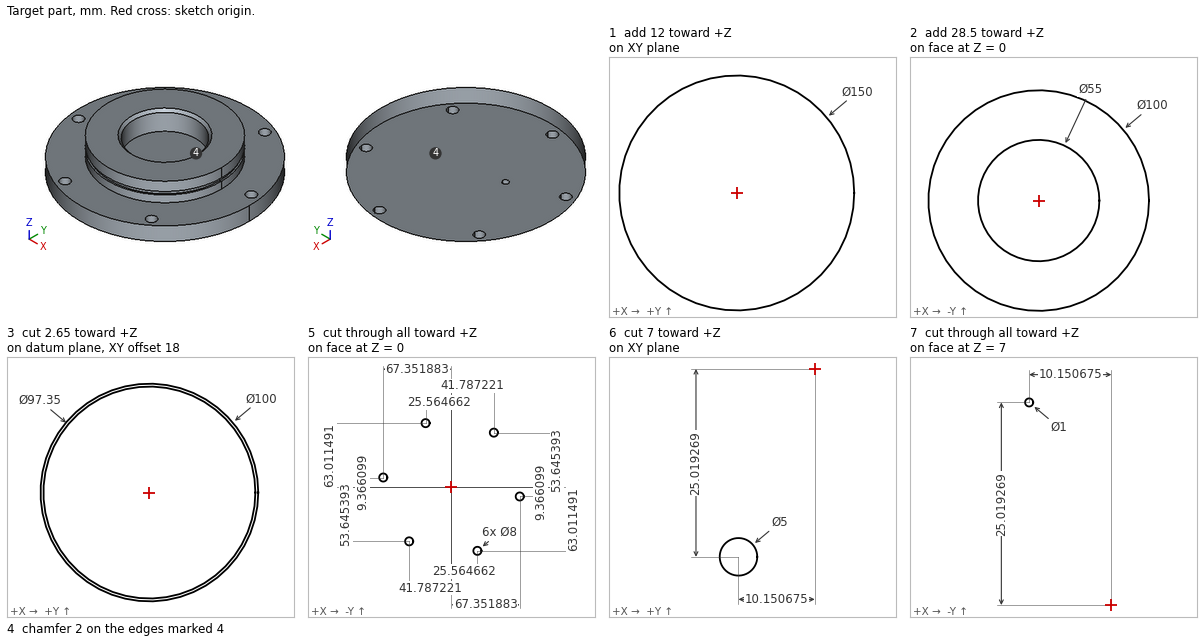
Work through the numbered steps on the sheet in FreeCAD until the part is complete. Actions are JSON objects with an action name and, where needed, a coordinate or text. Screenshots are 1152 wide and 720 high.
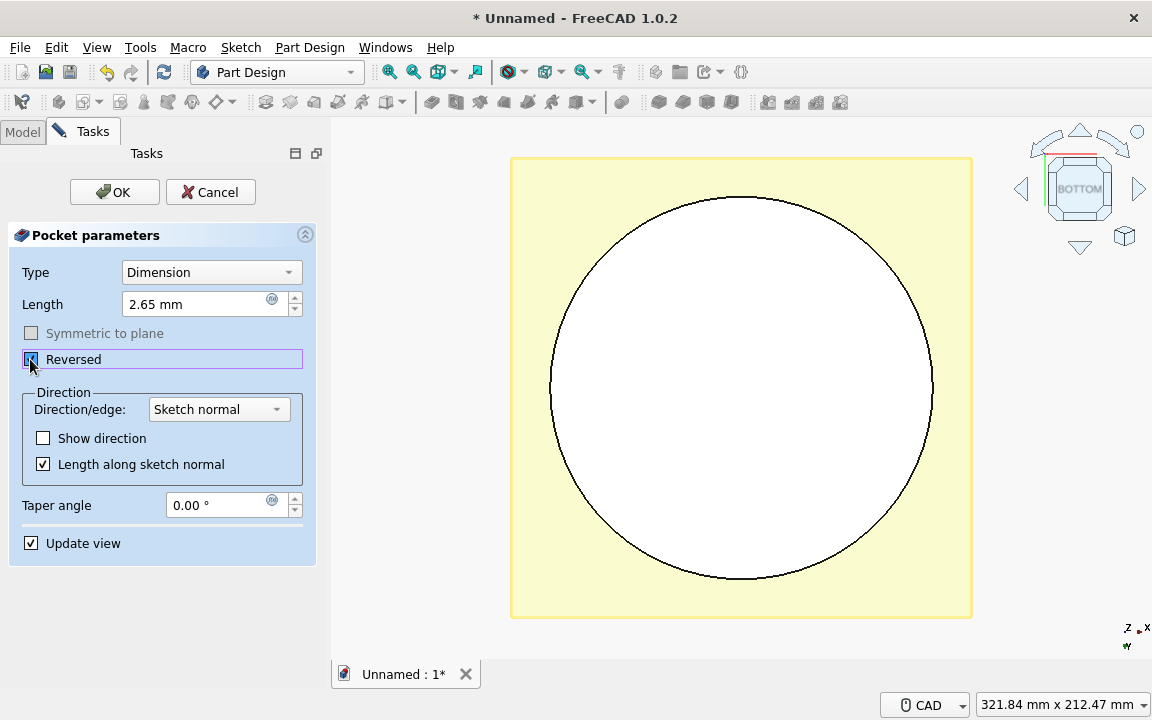
{"action": "left_click", "coordinate": [115, 192]}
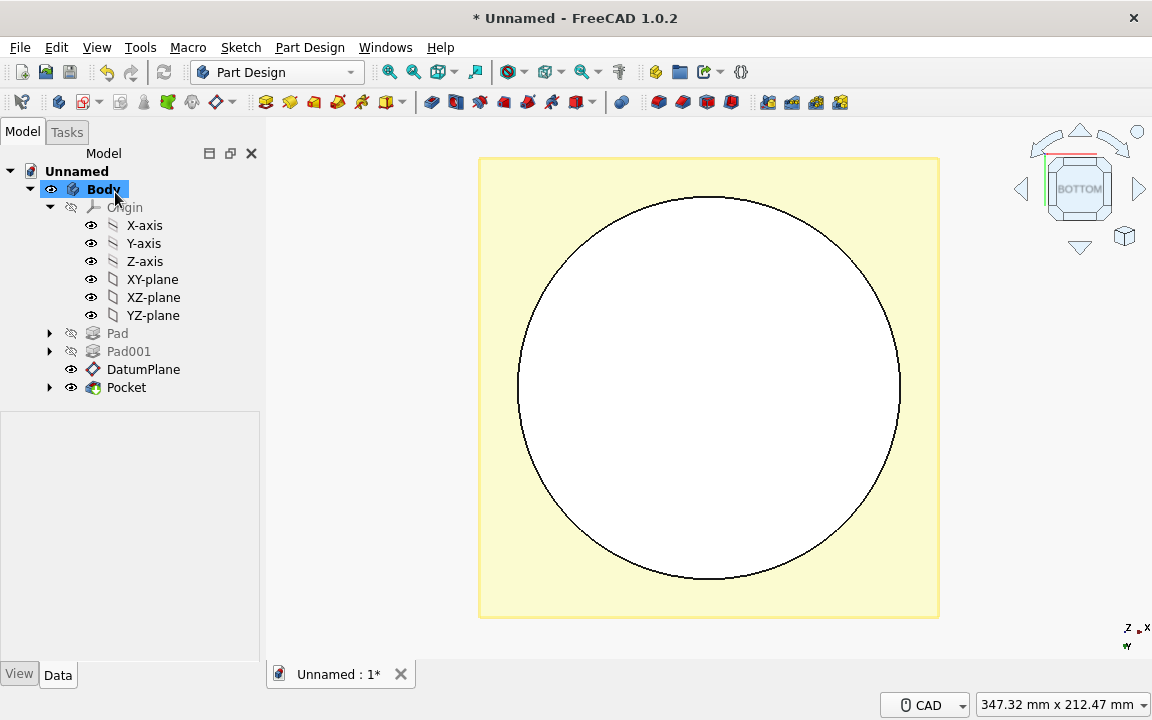
{"action": "left_click", "coordinate": [116, 369]}
{"action": "key", "text": "space"}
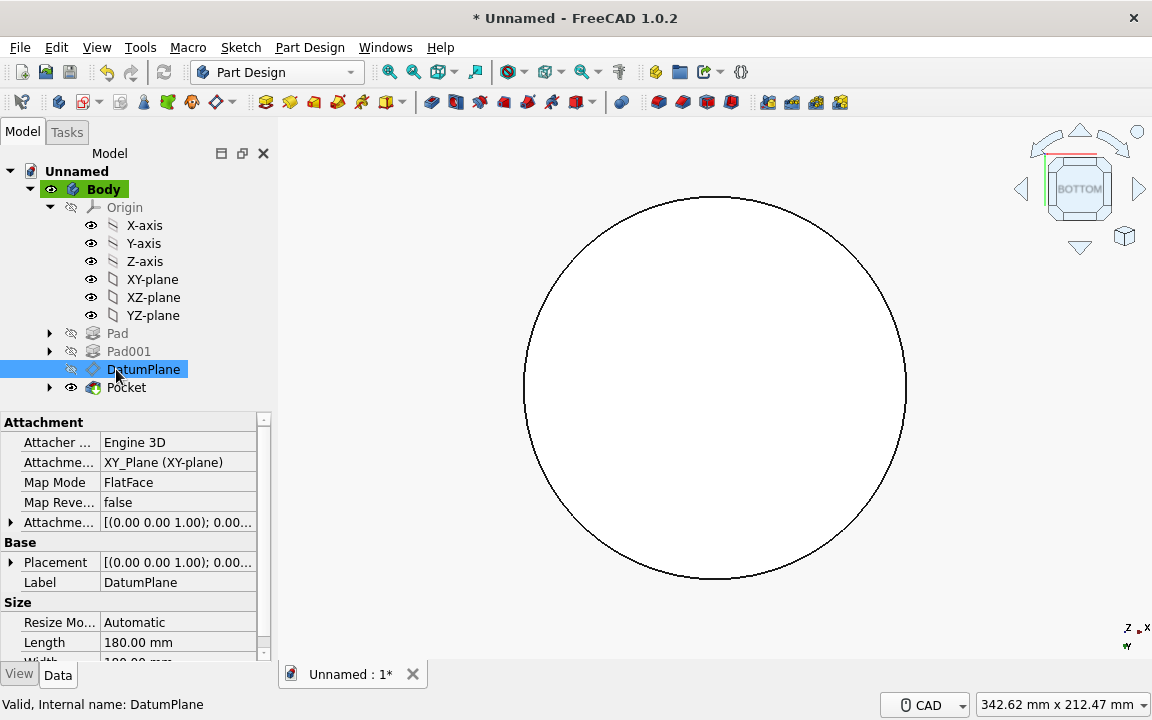
{"action": "key", "text": "0"}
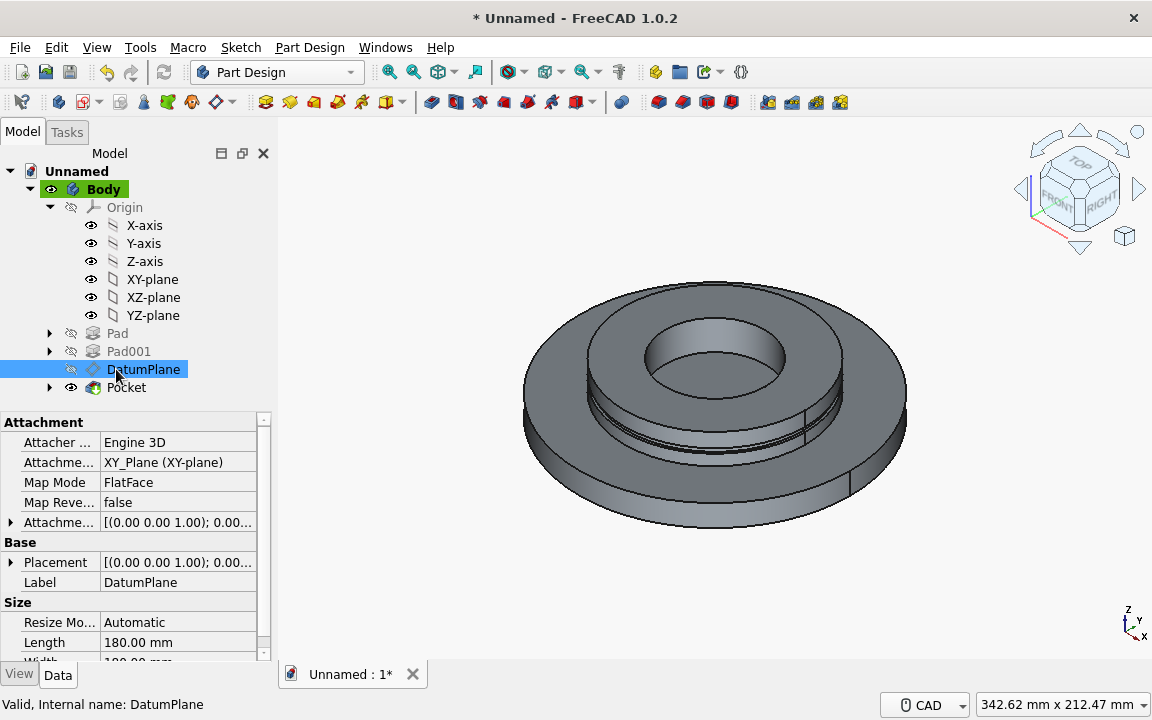
{"action": "left_click", "coordinate": [665, 329]}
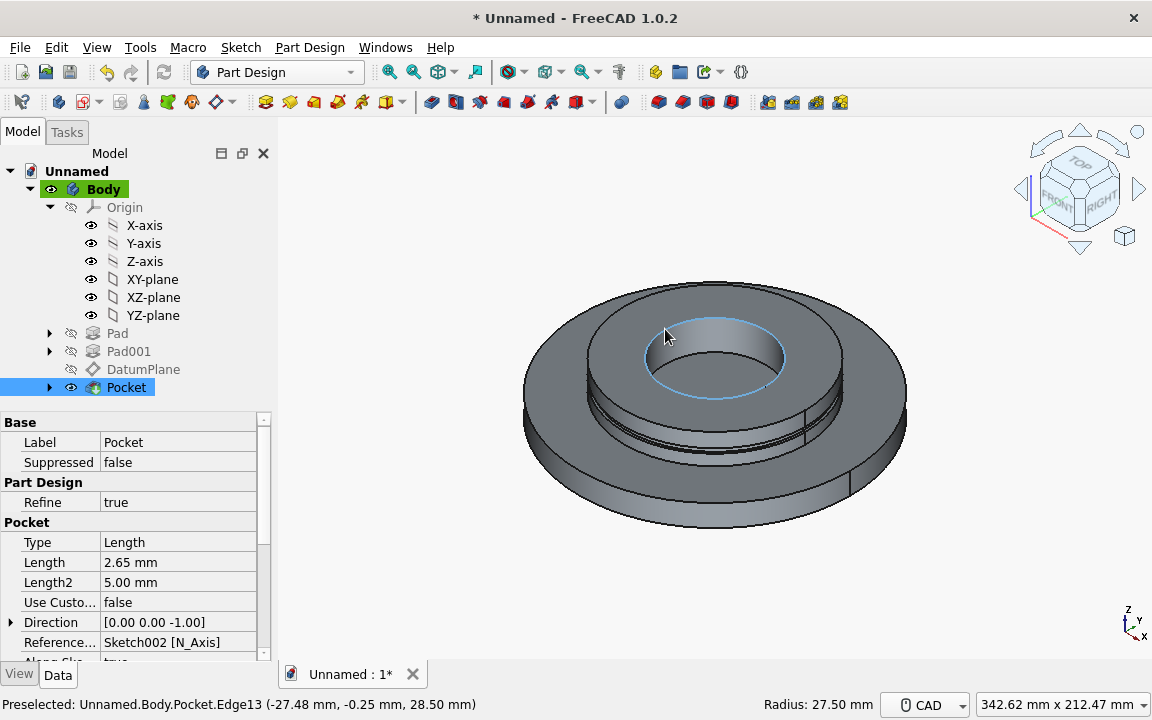
{"action": "left_click", "coordinate": [684, 102]}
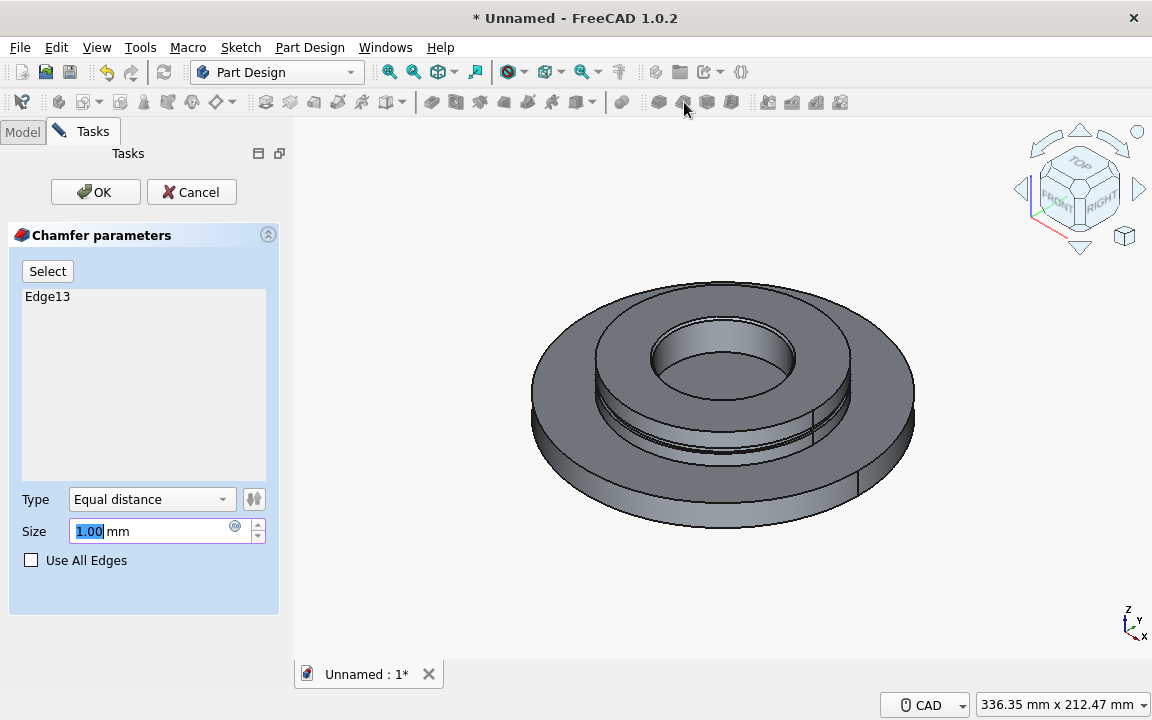
{"action": "type", "text": "2"}
{"action": "key", "text": "Tab"}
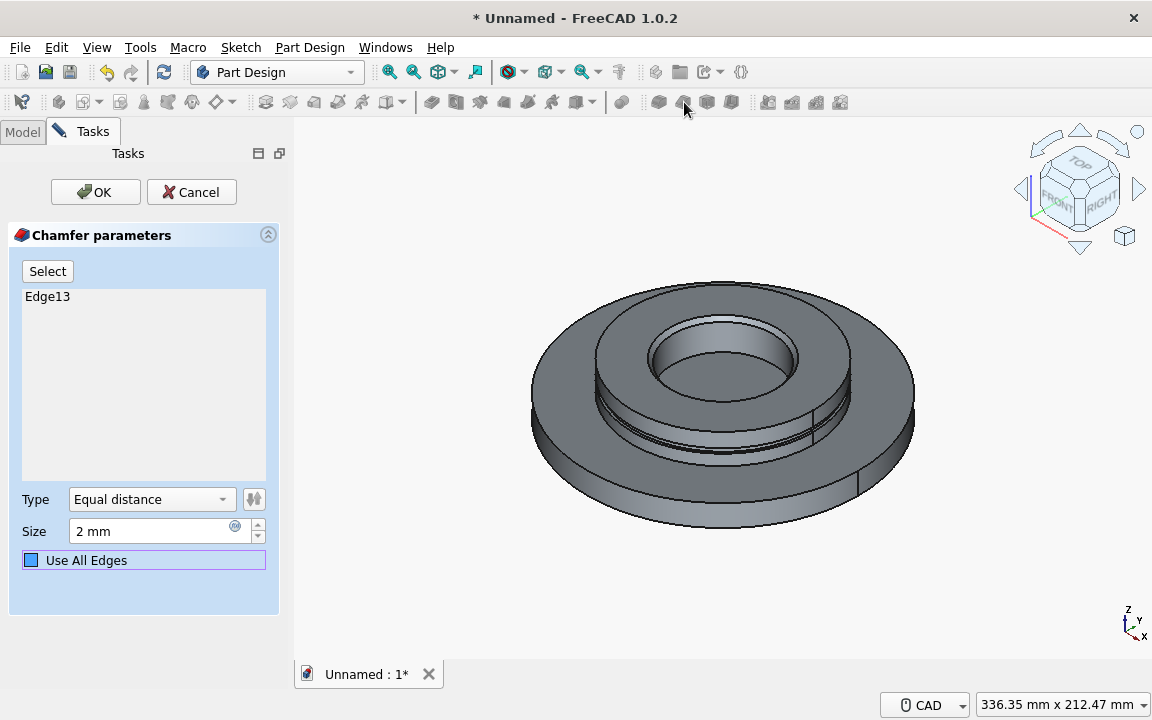
{"action": "left_click", "coordinate": [96, 192]}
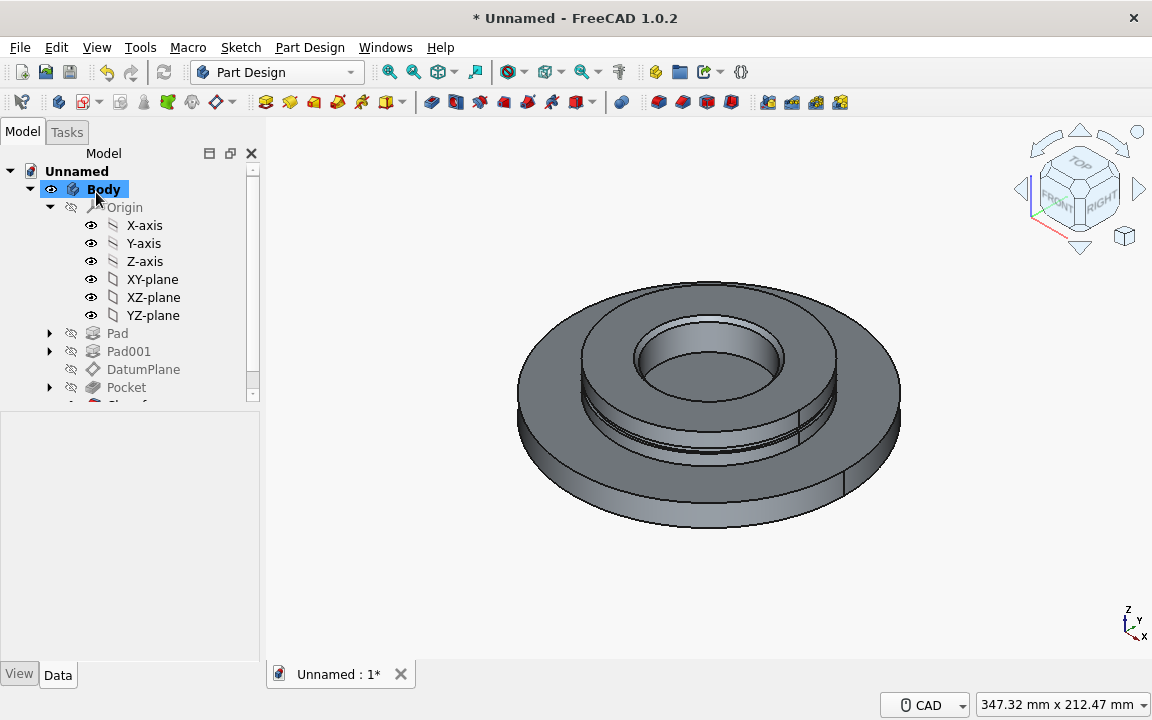
{"action": "key", "text": "5"}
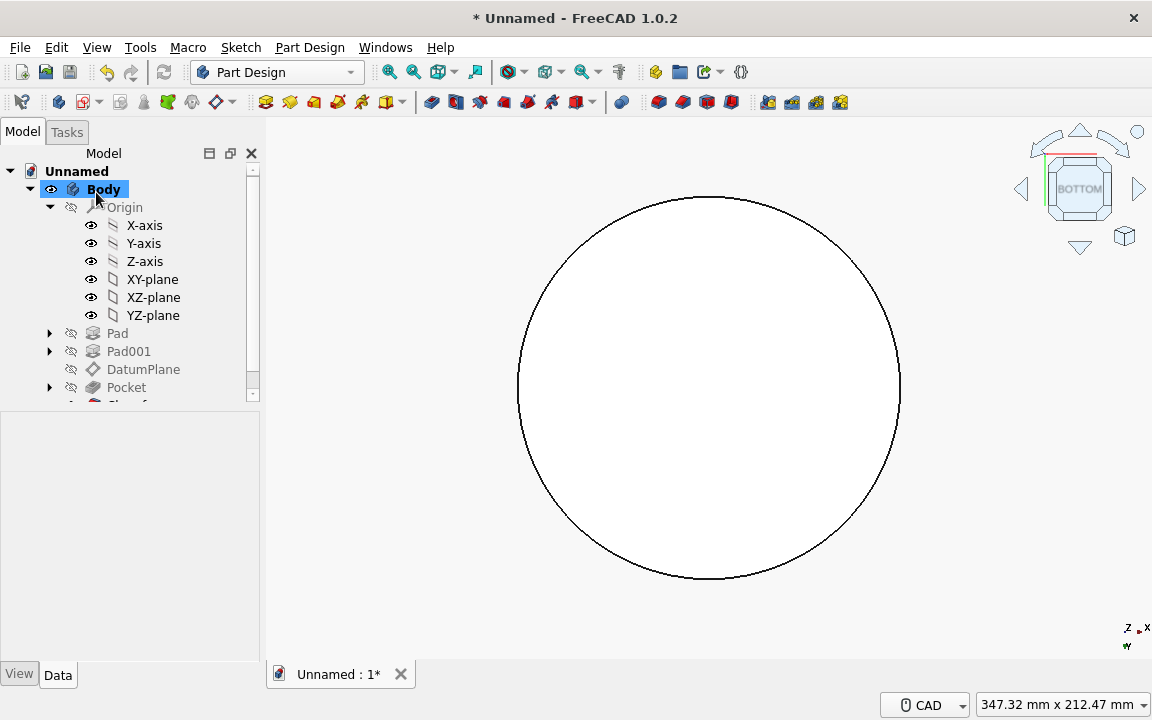
{"action": "left_click", "coordinate": [709, 387]}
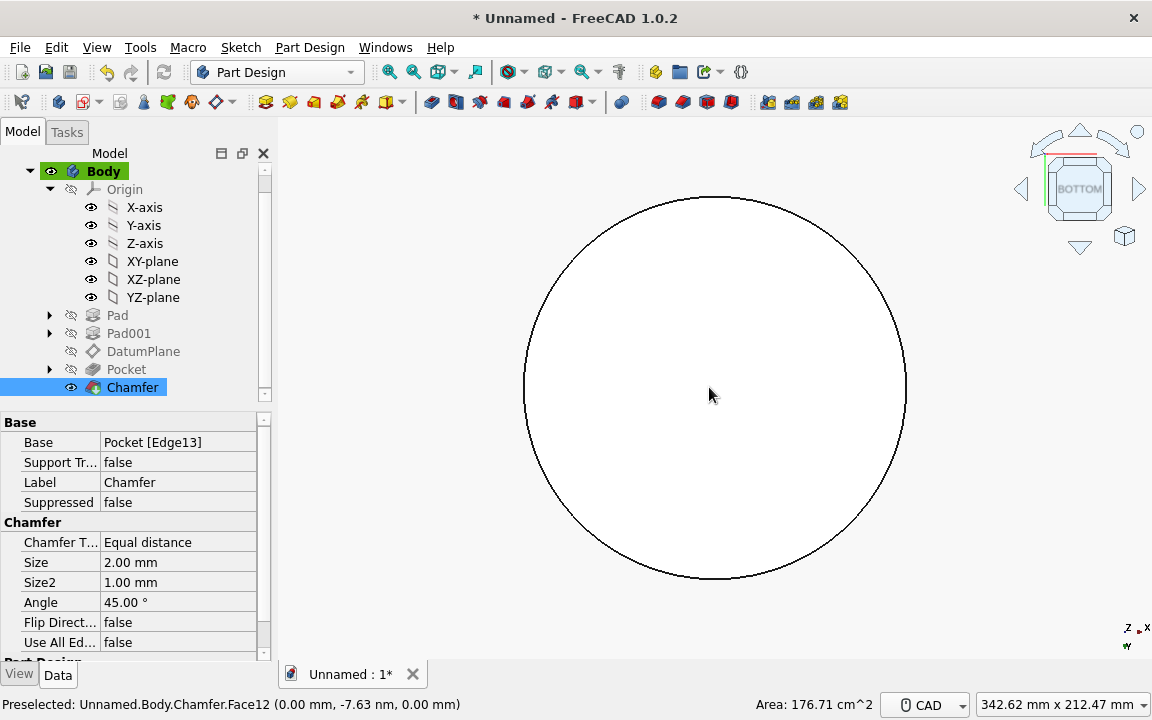
{"action": "left_click", "coordinate": [84, 102]}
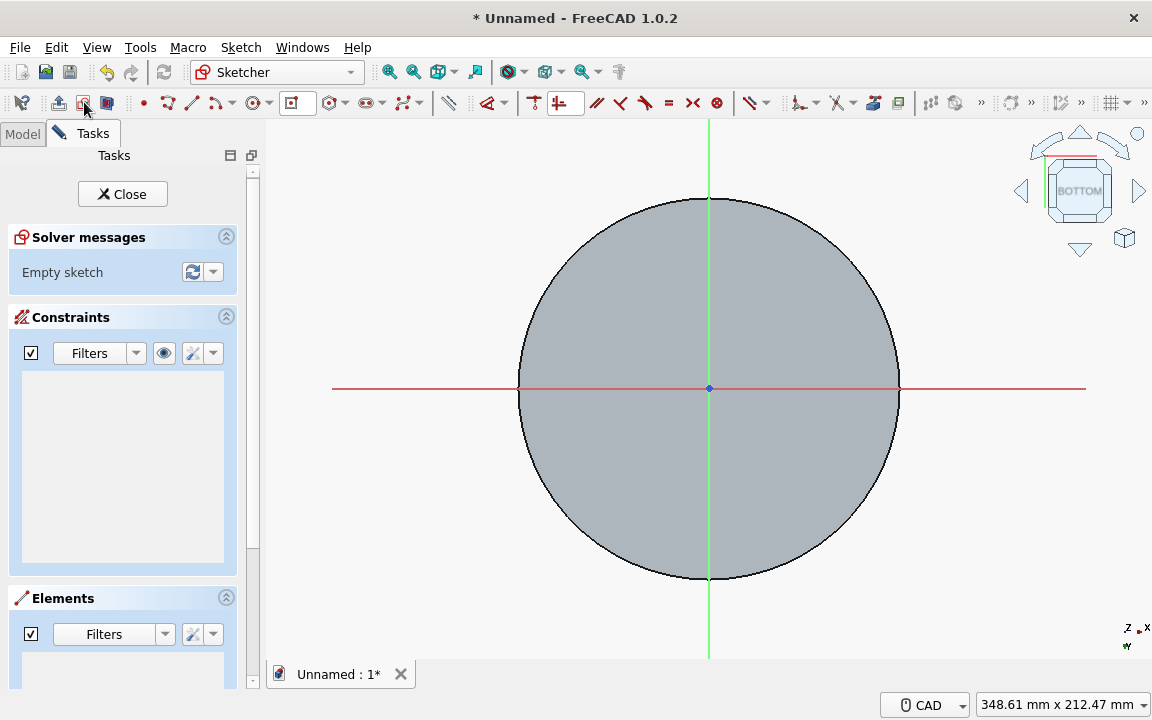
{"action": "left_click", "coordinate": [254, 104]}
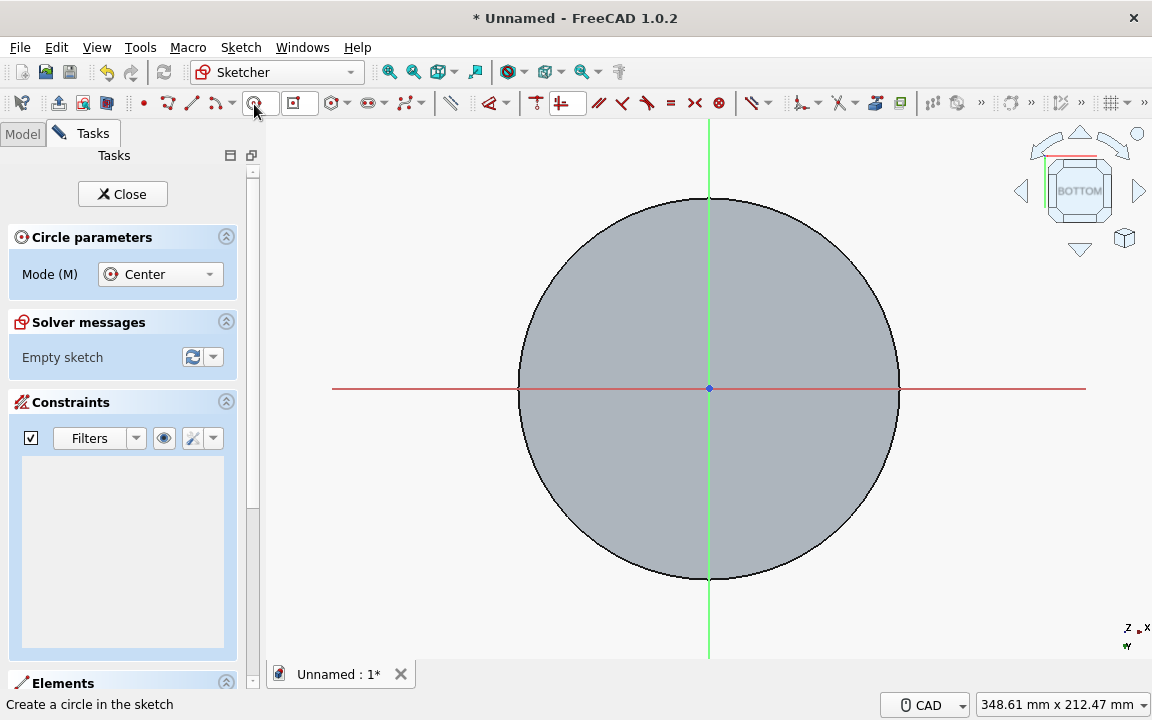
{"action": "scroll", "coordinate": [774, 549], "scroll_direction": "up", "scroll_amount": 5}